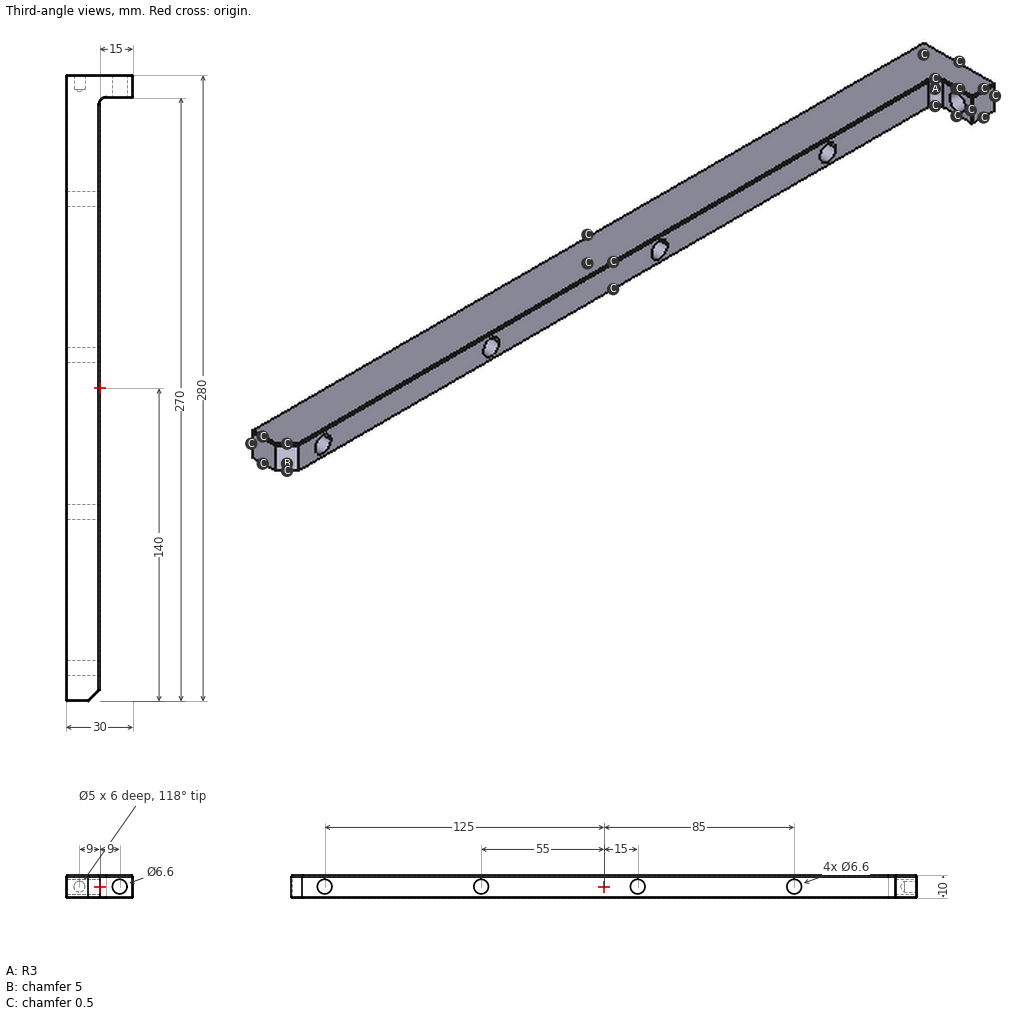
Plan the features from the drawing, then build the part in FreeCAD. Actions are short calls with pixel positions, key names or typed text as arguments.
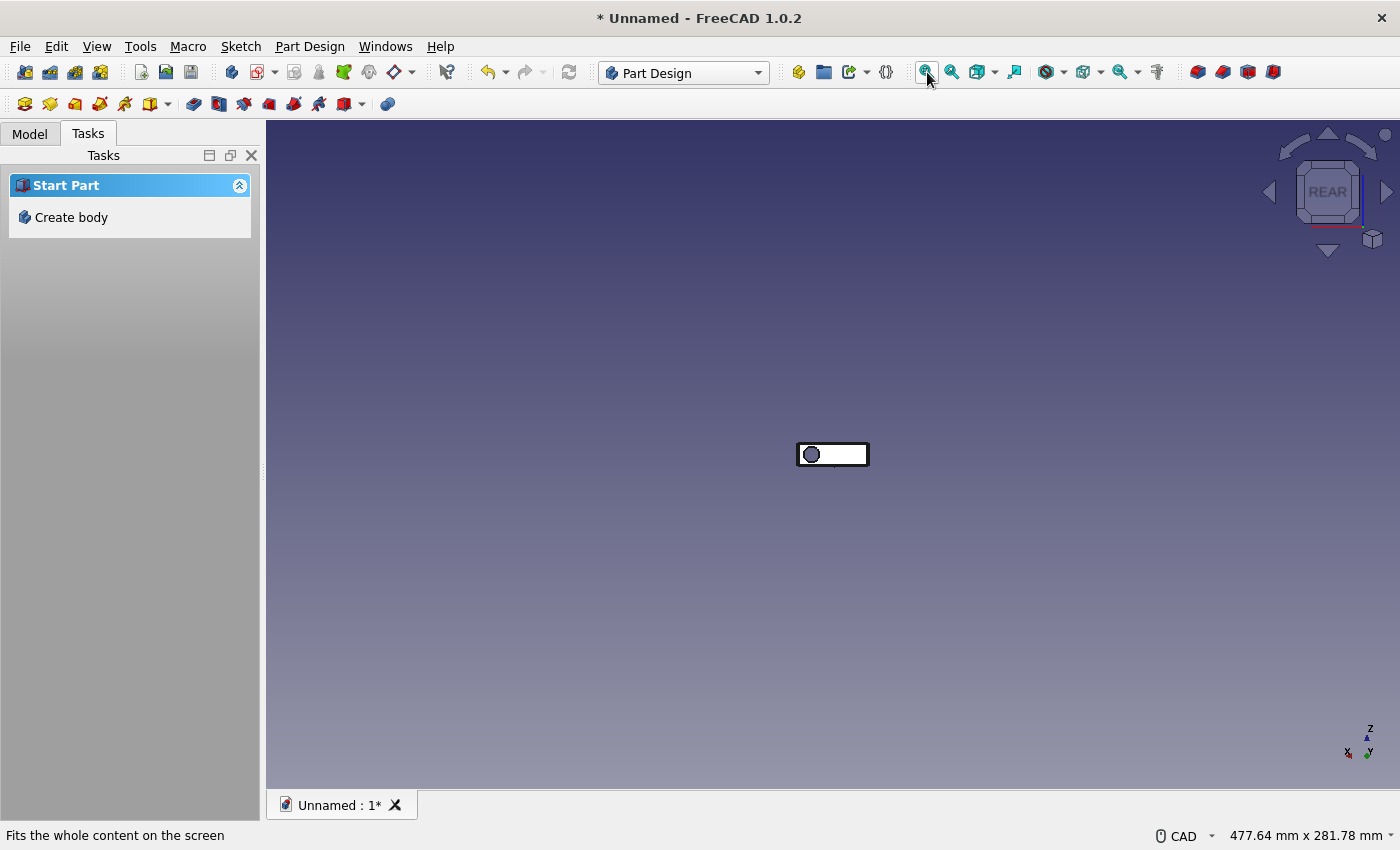
click(833, 454)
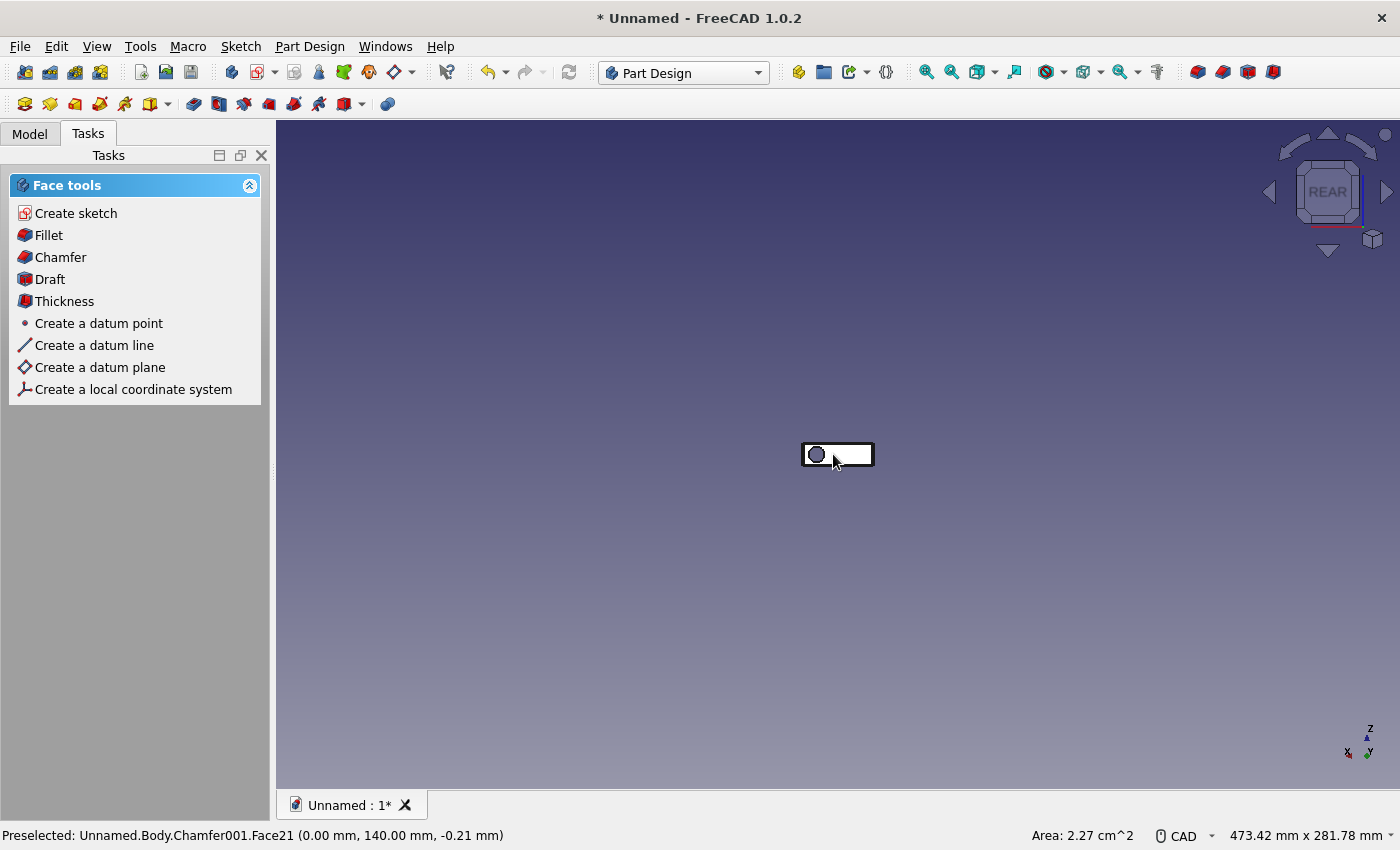
click(256, 72)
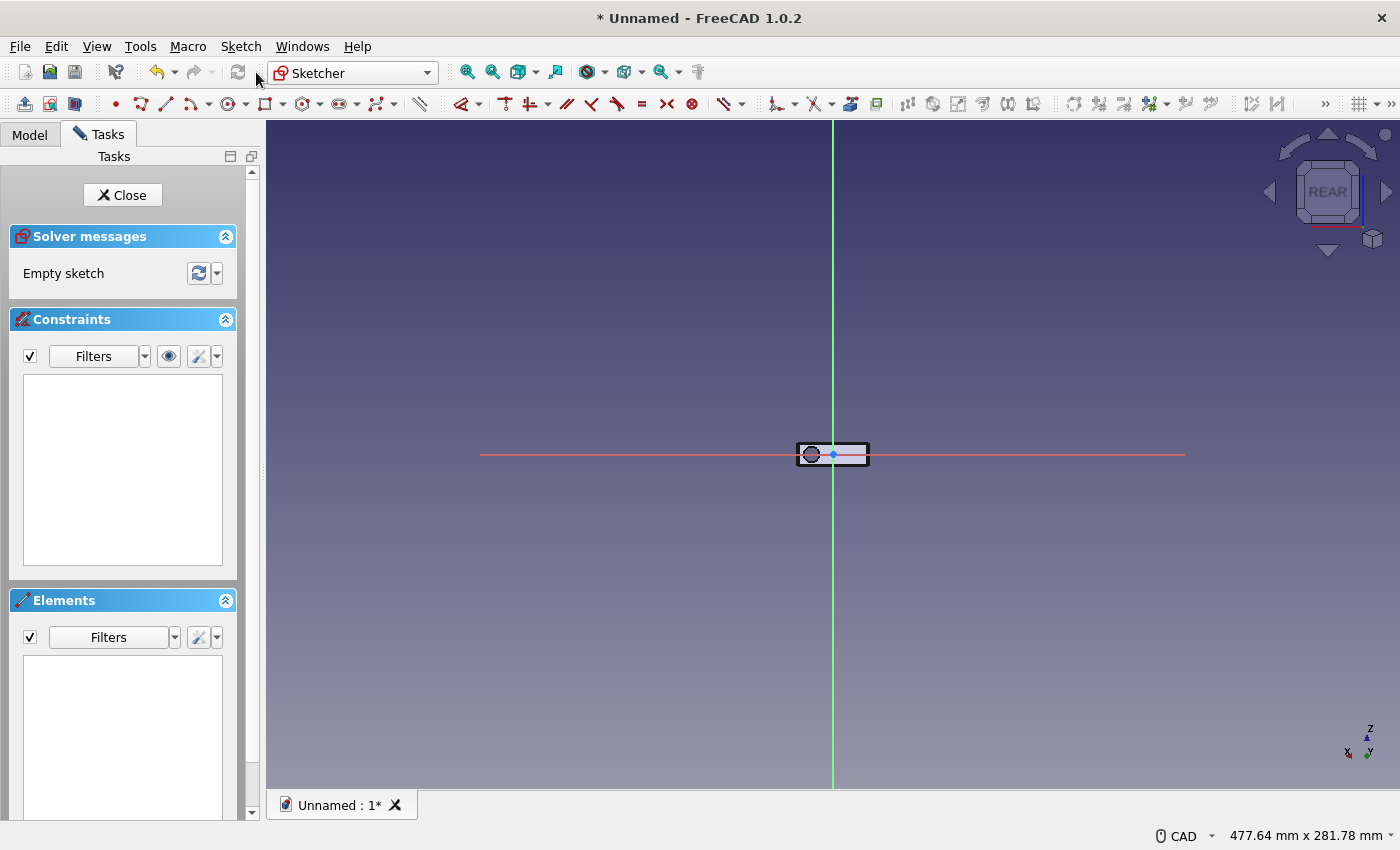
scroll(851, 455, up, 15)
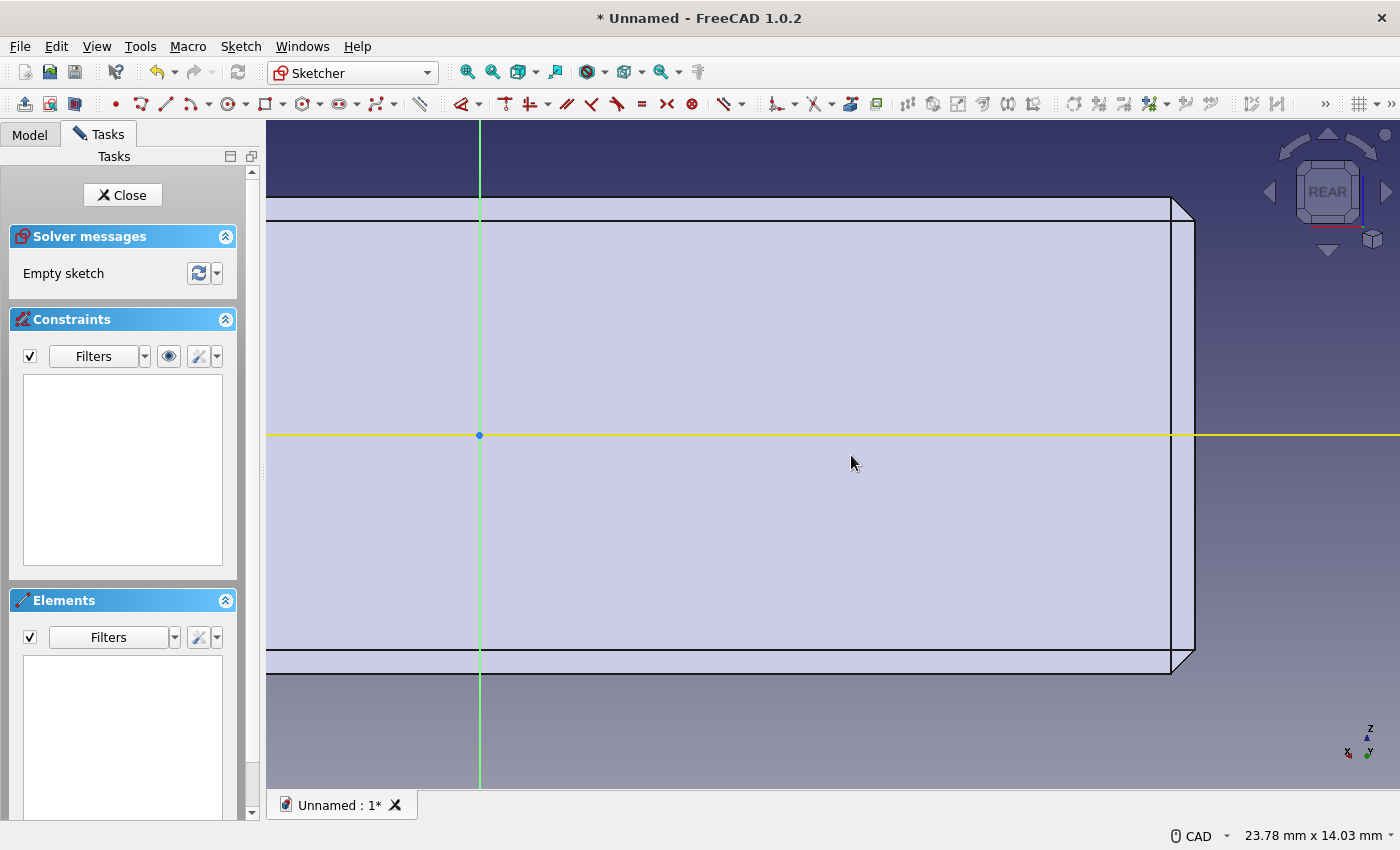
click(228, 104)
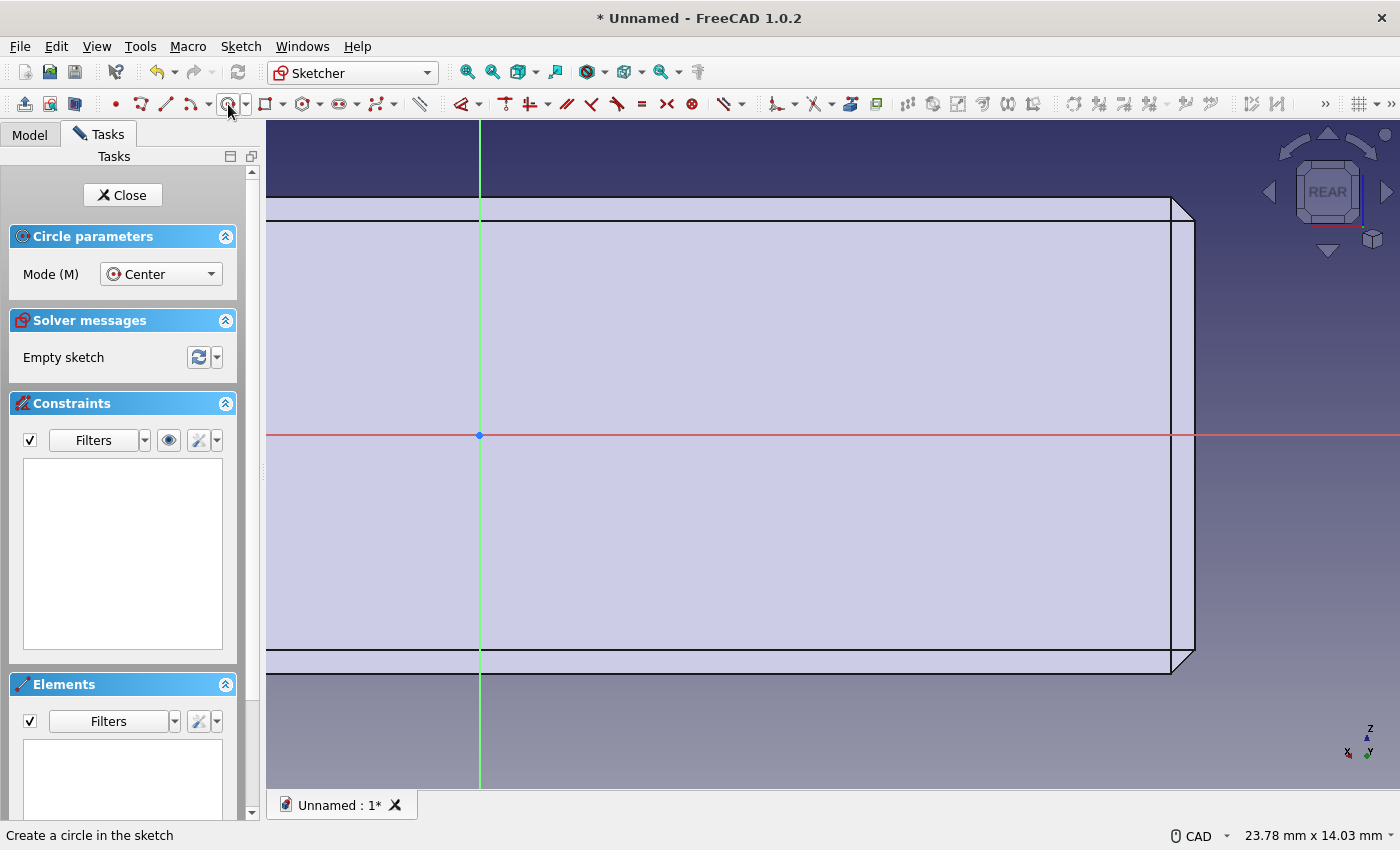
click(909, 435)
click(993, 351)
key(Escape)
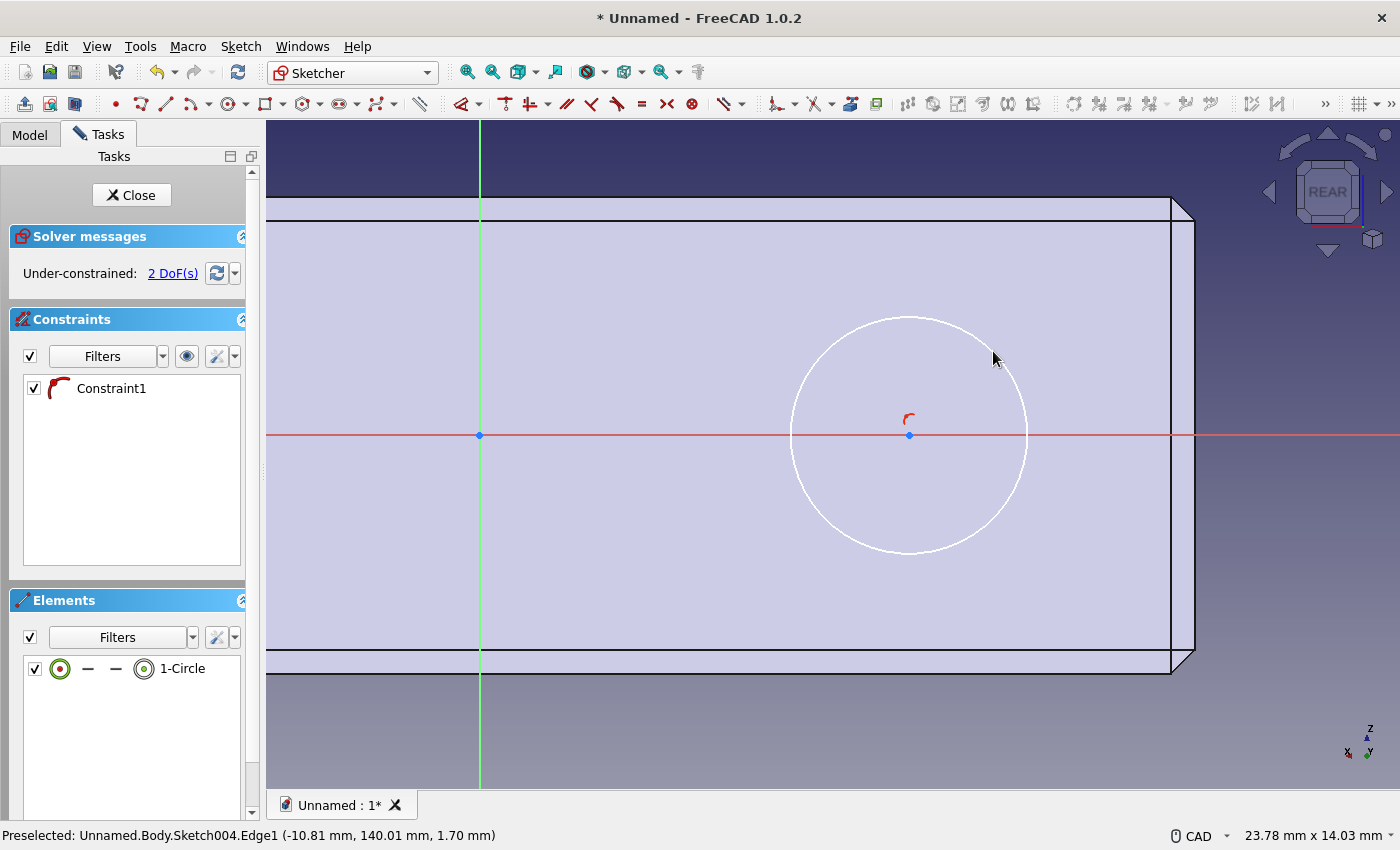
click(460, 104)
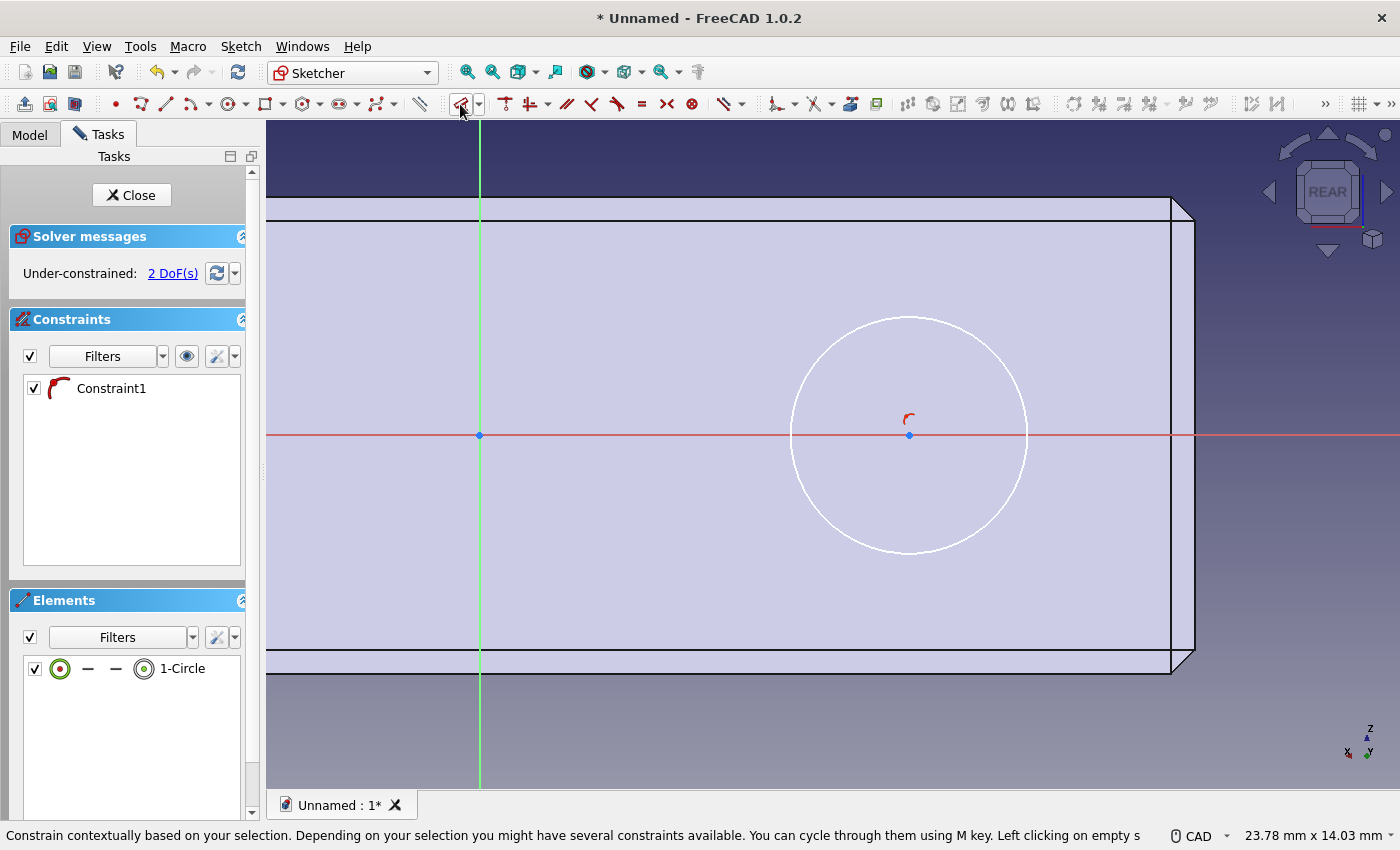
click(992, 351)
click(1014, 328)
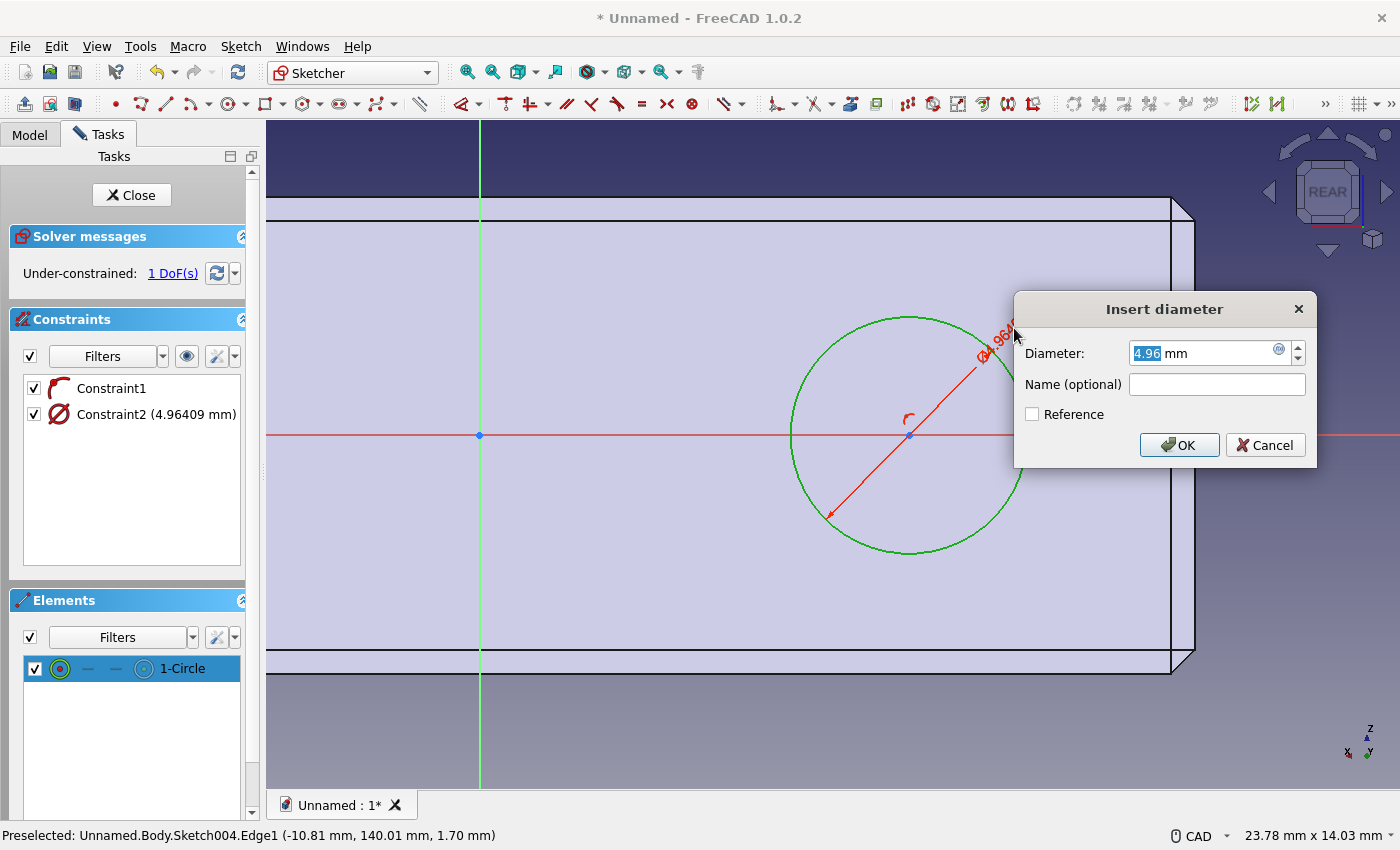
text(5)
key(Return)